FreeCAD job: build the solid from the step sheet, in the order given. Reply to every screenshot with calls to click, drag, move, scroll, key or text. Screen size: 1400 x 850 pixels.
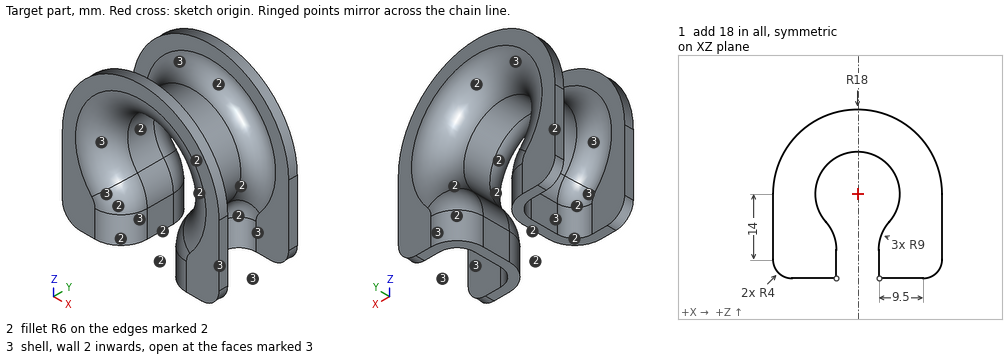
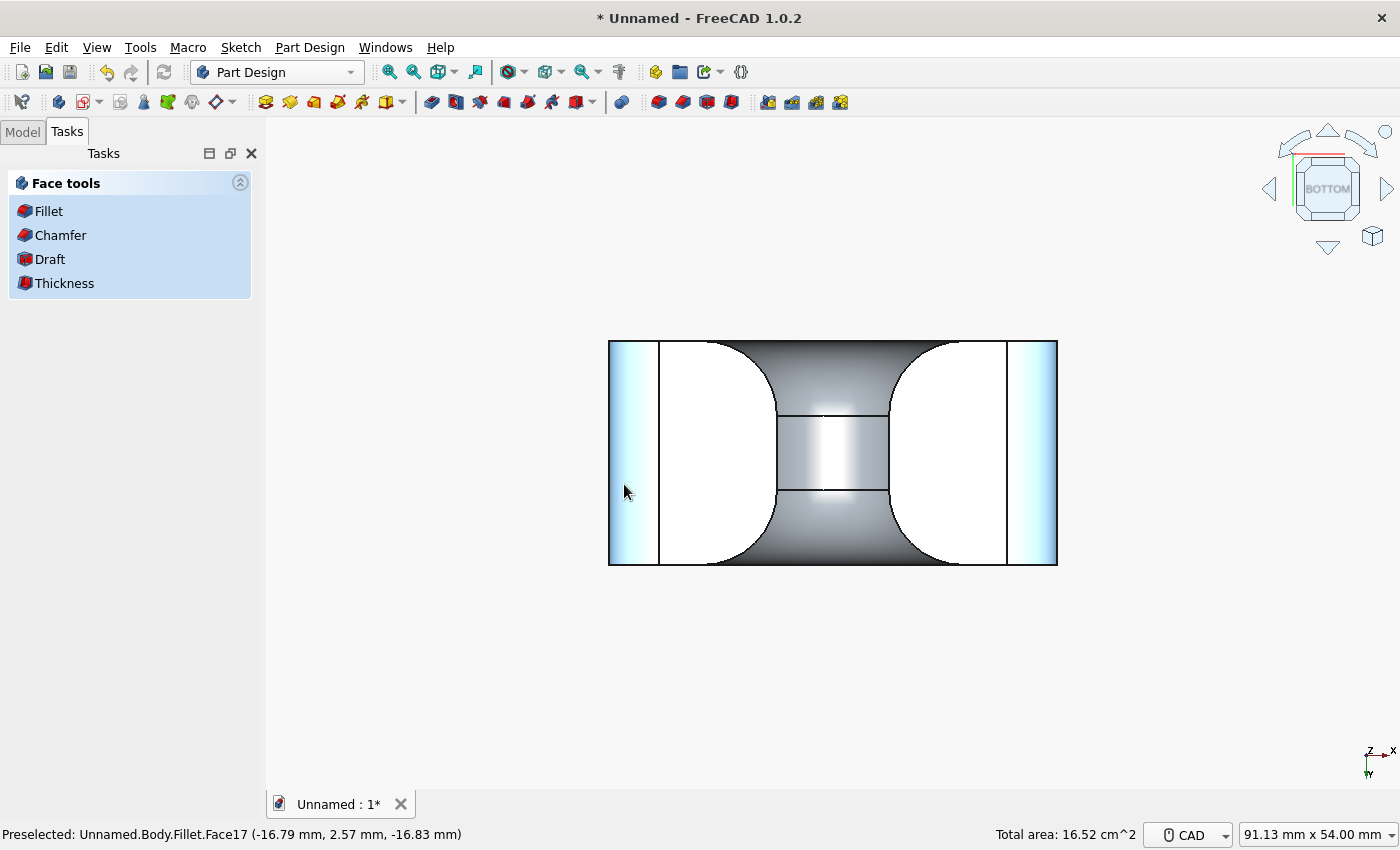
click(948, 484, ctrl)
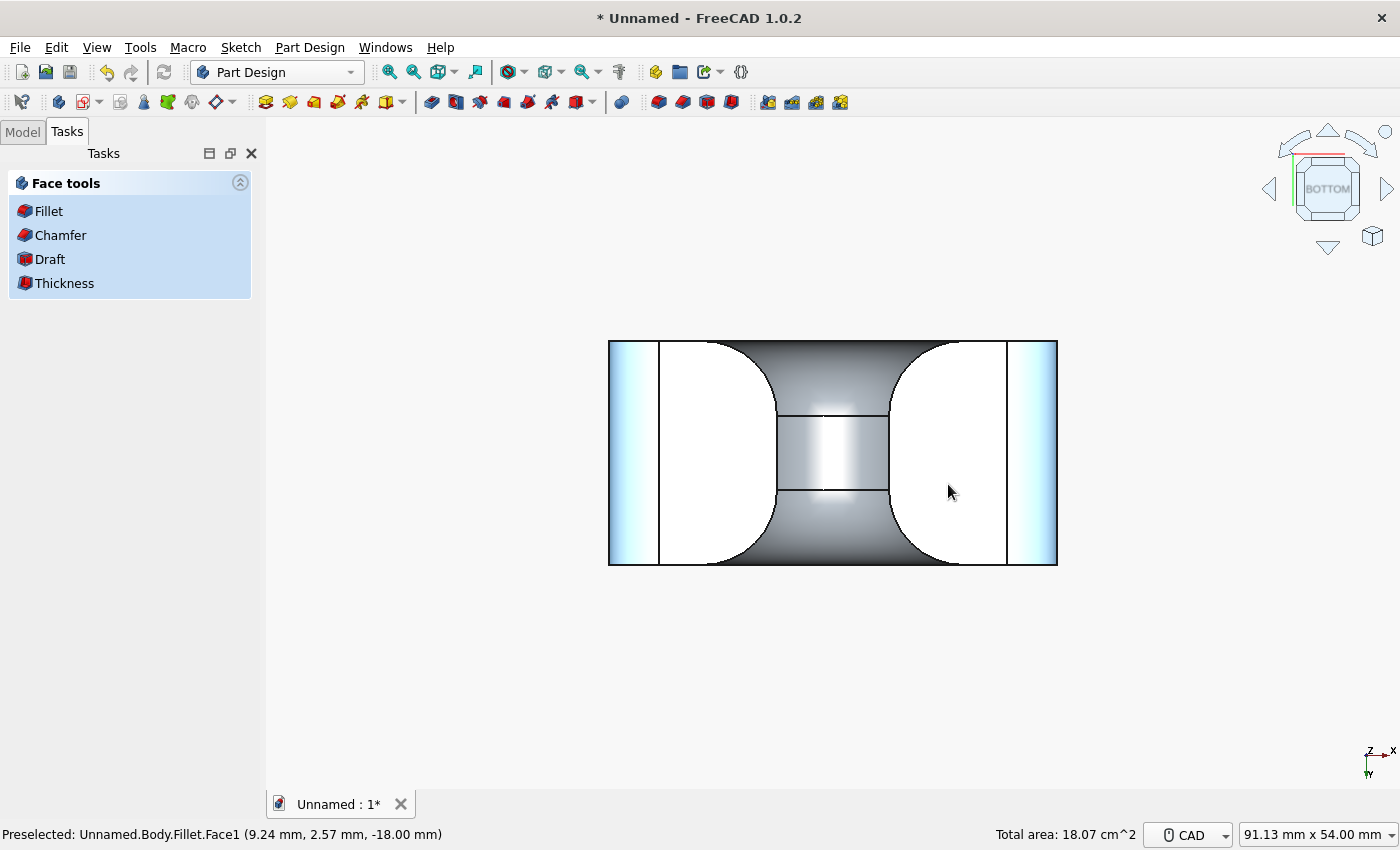
key(4)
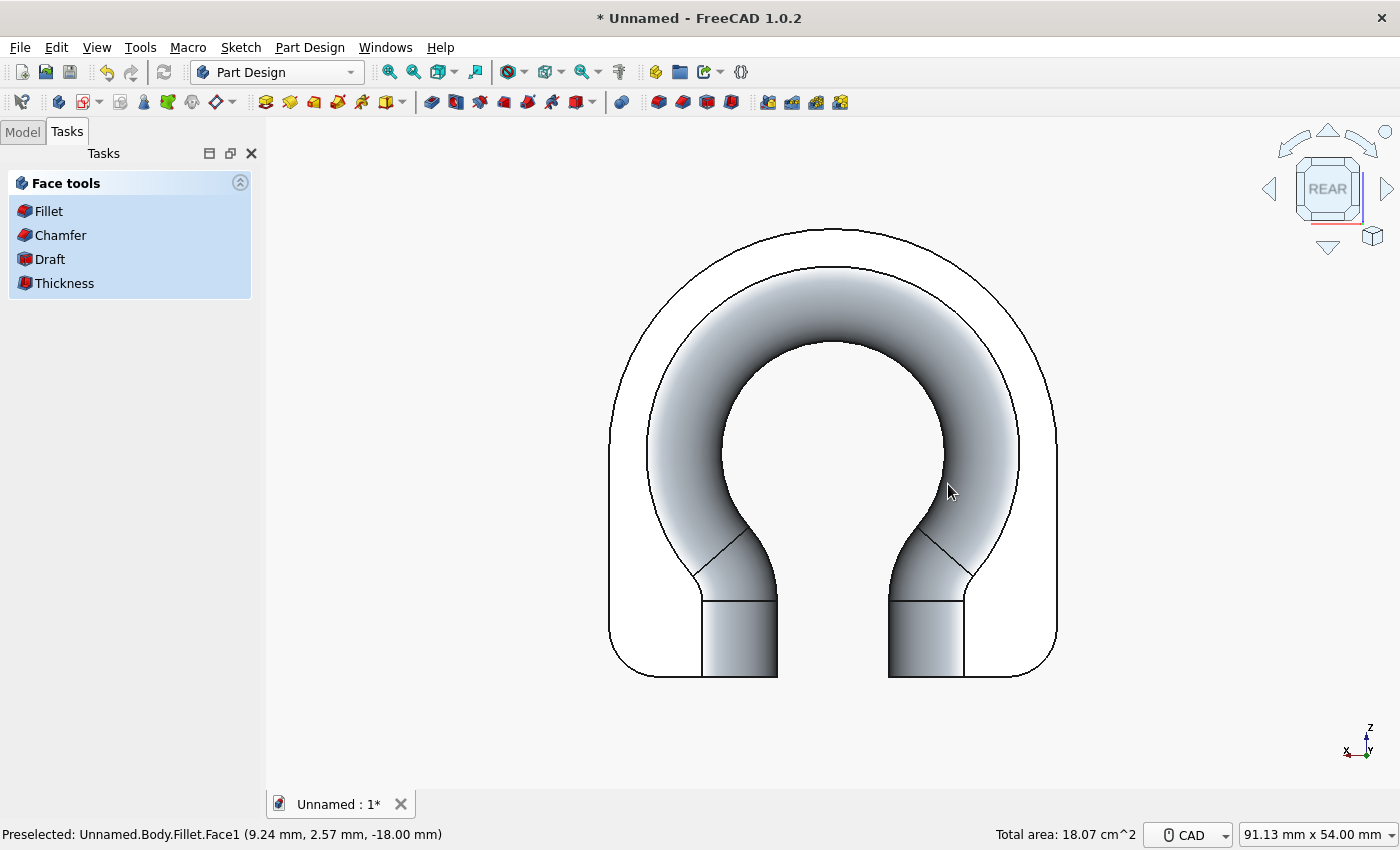
key(6)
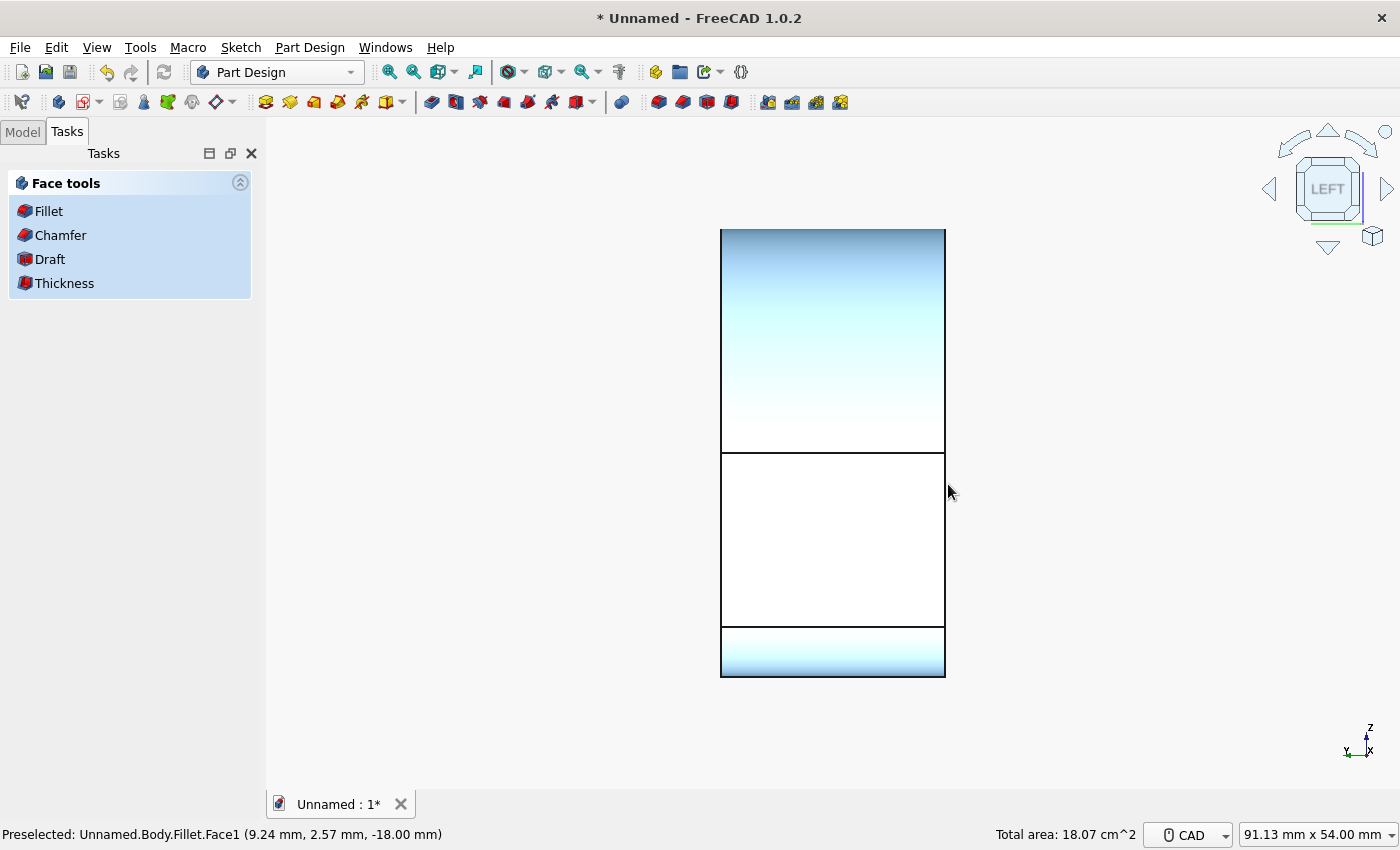
click(833, 539, ctrl)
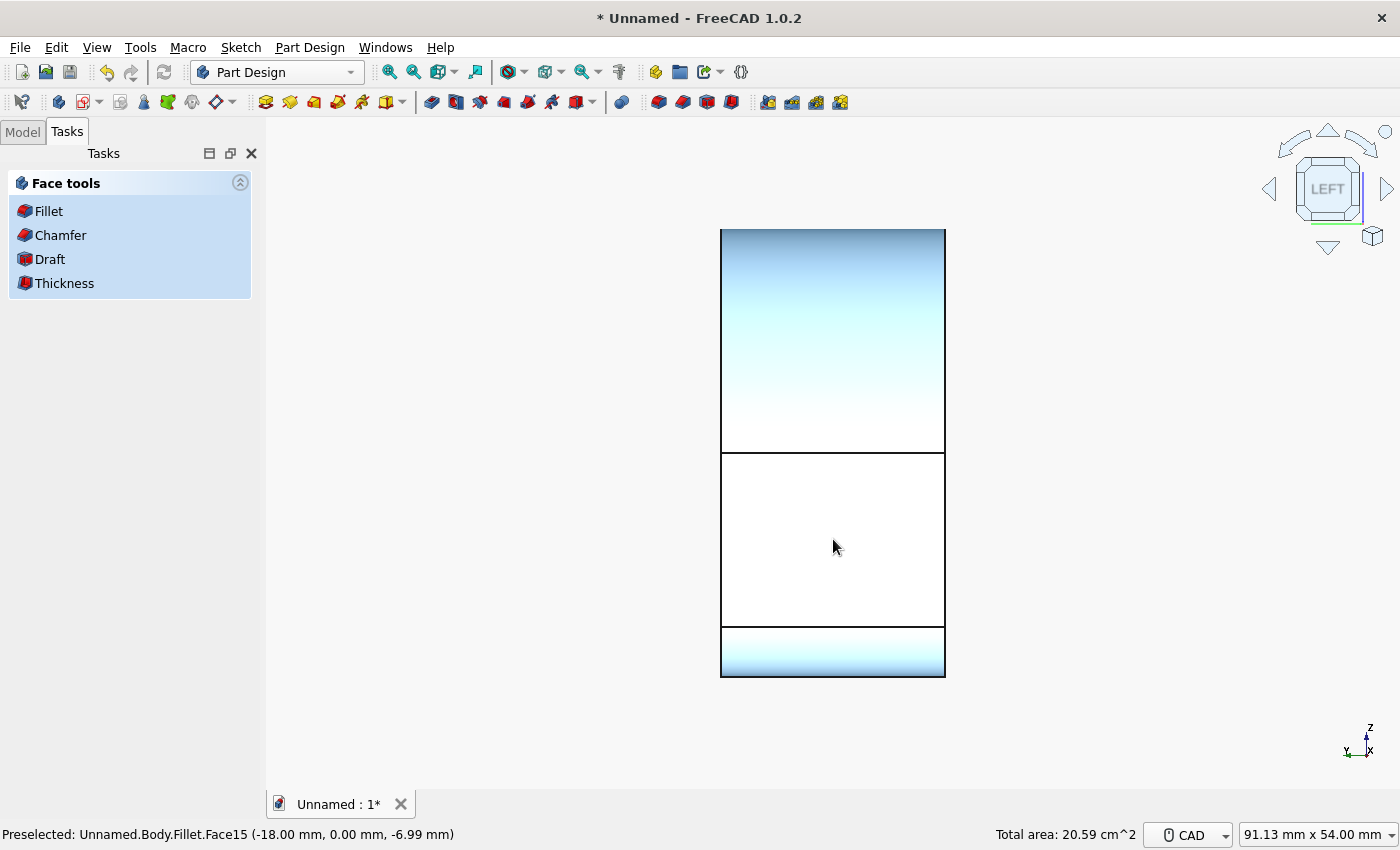
click(732, 102)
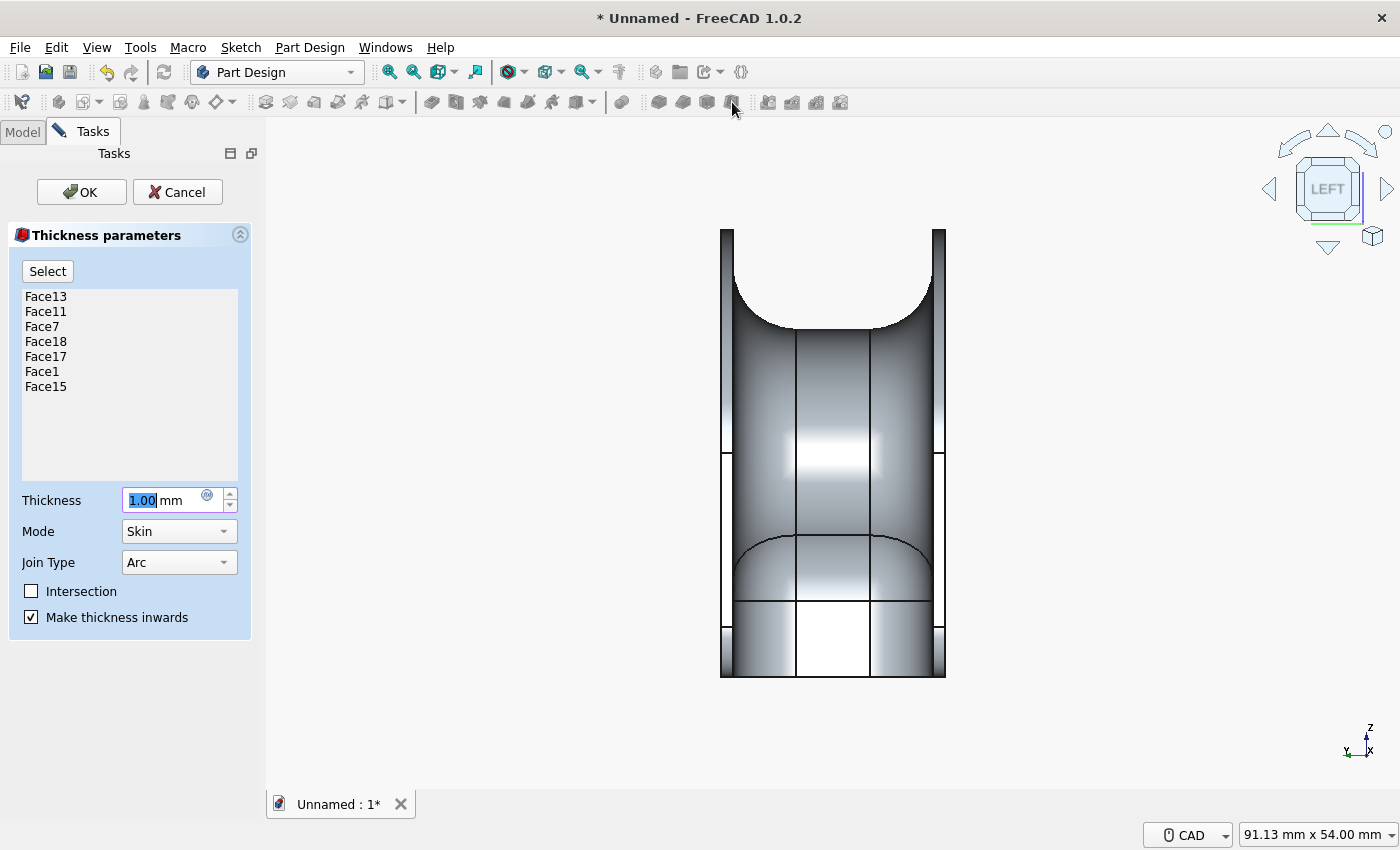
text(2)
key(Tab)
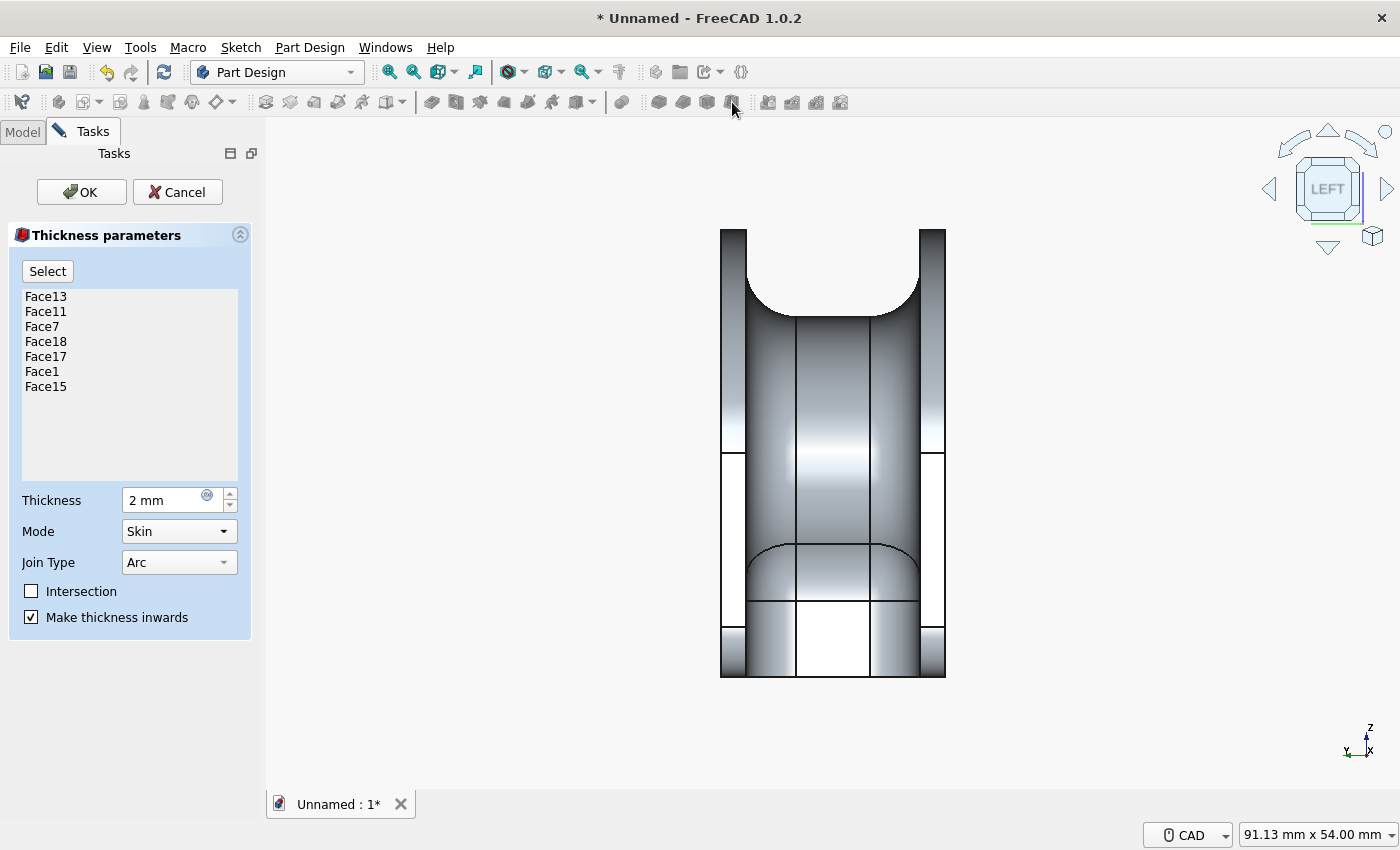
click(180, 562)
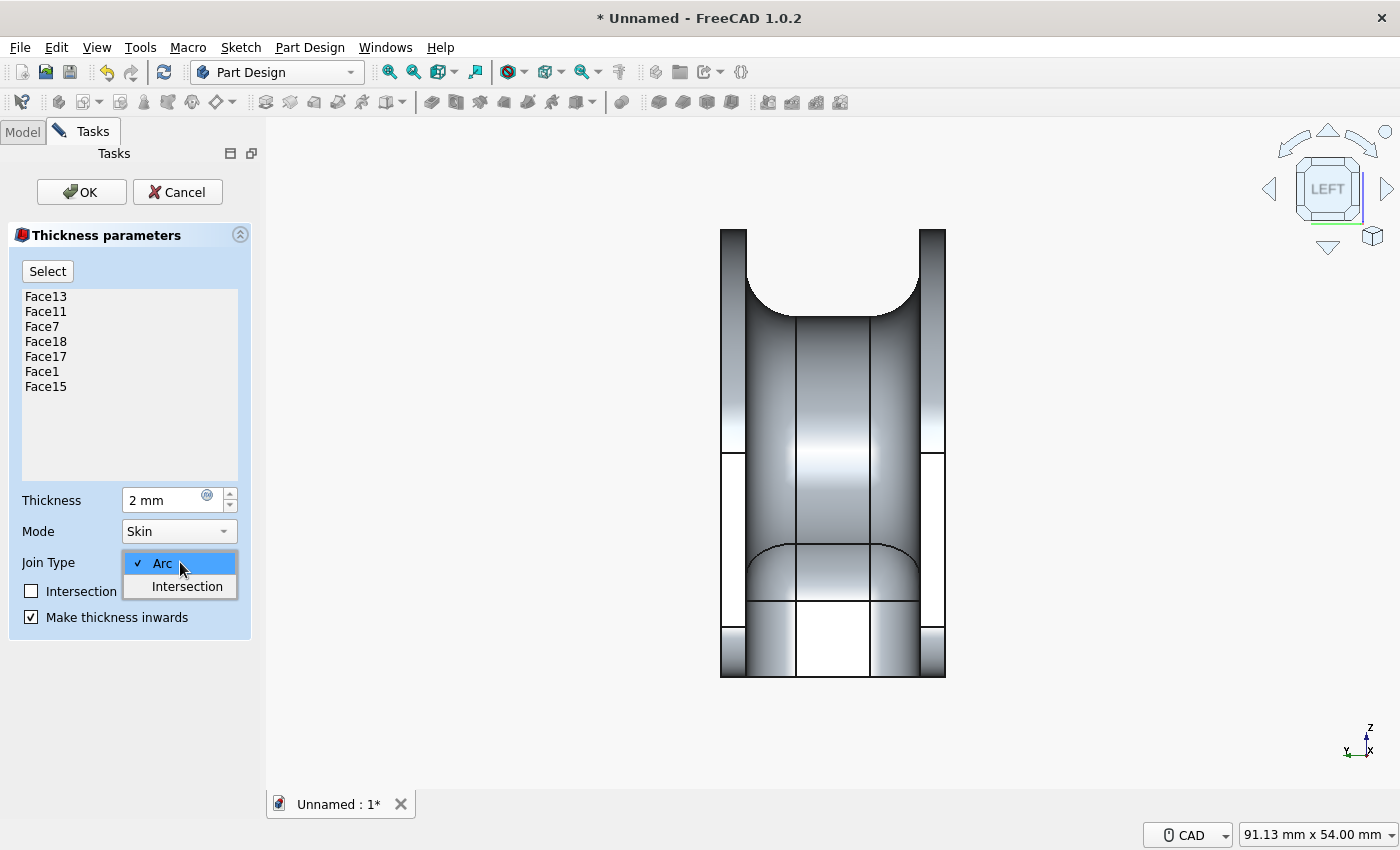
click(179, 586)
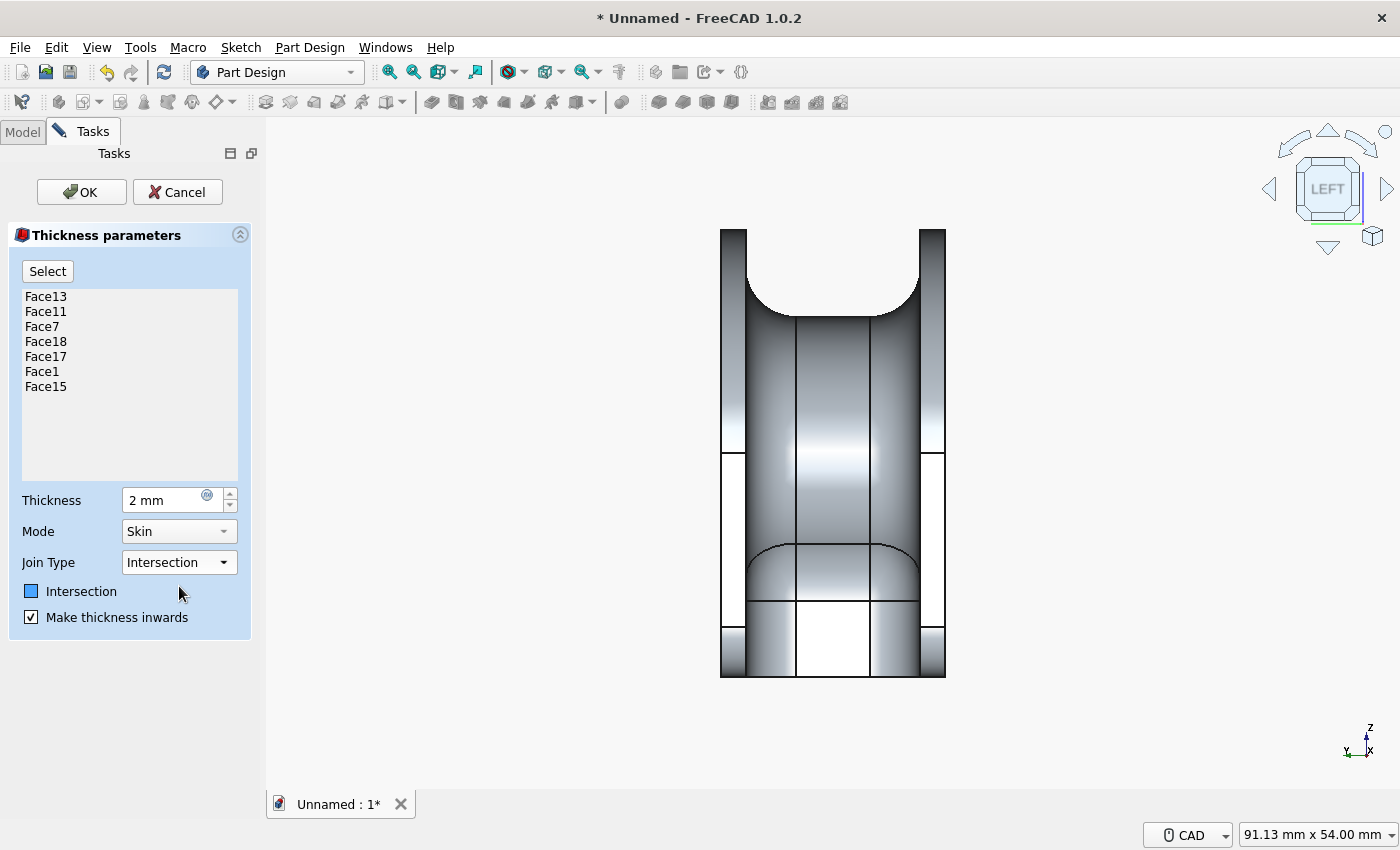
click(82, 192)